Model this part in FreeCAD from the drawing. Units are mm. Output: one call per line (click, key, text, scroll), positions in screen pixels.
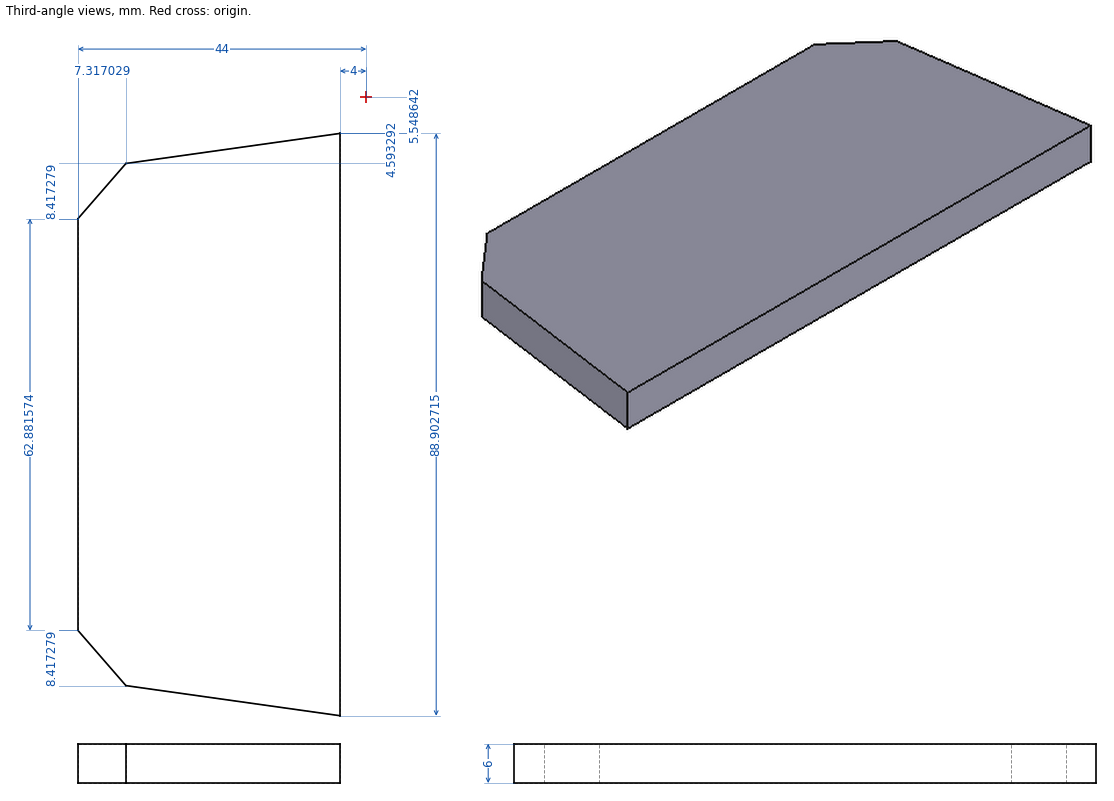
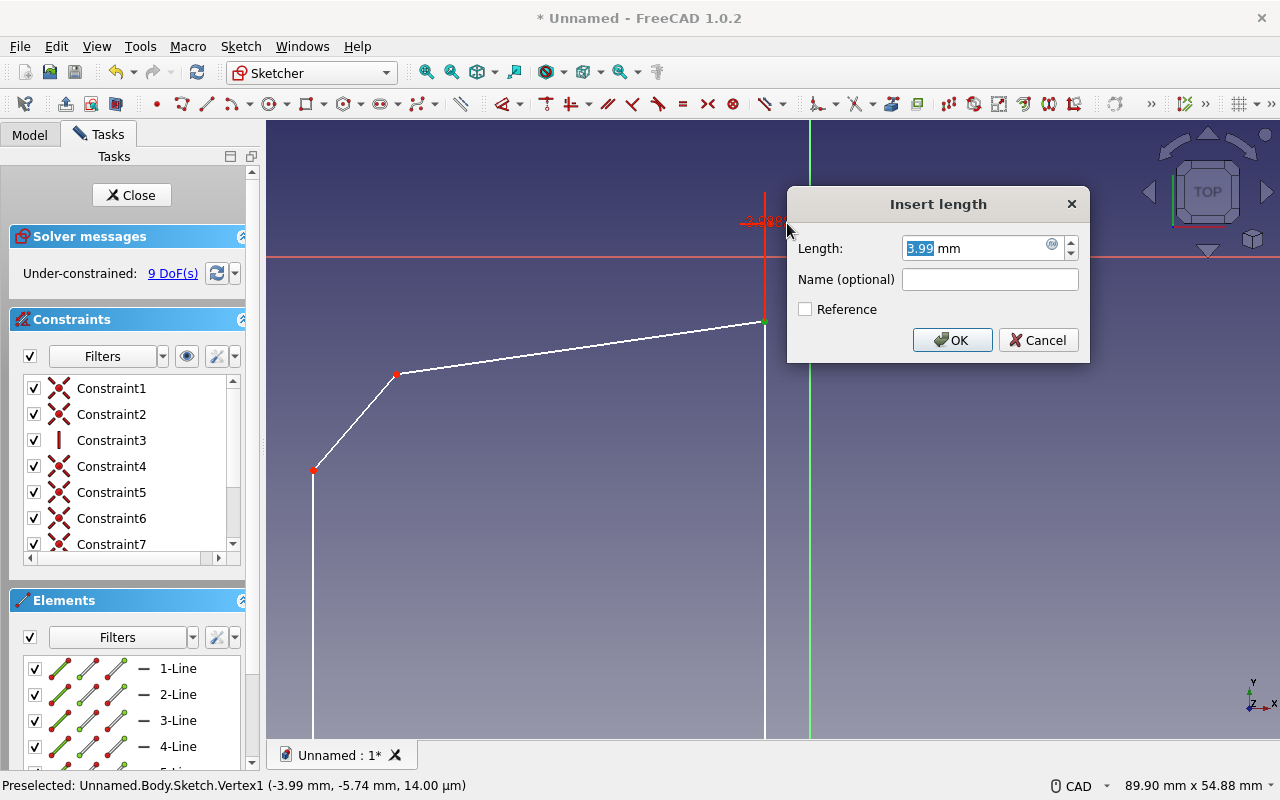
text(4)
key(Return)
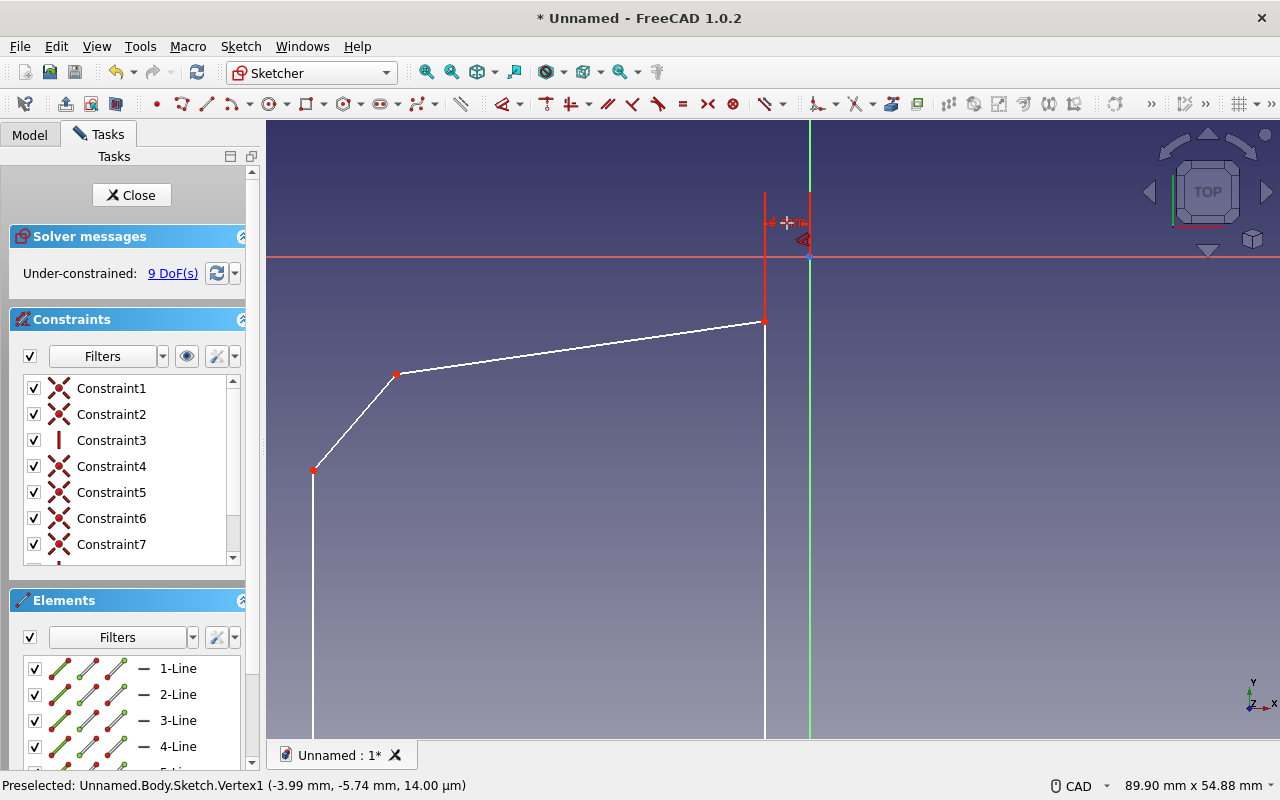
click(313, 471)
click(562, 223)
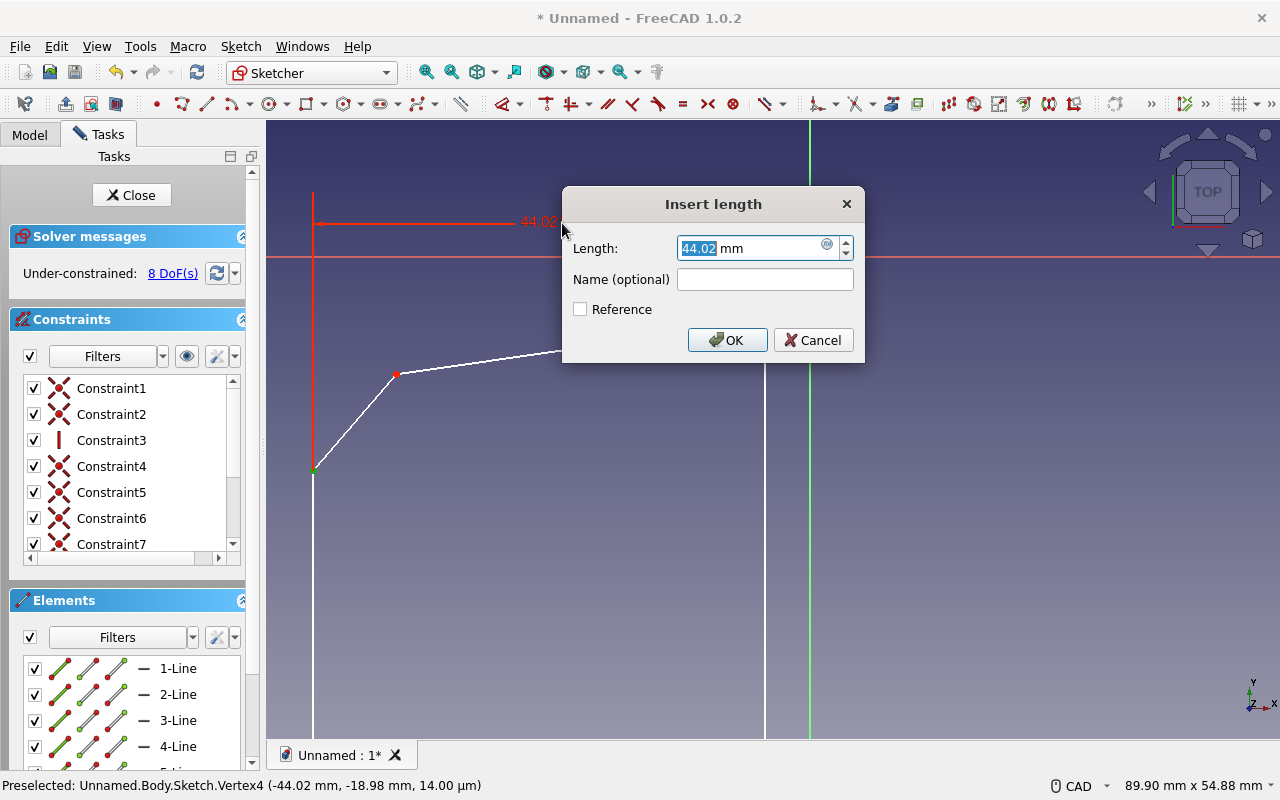
text(44)
key(Return)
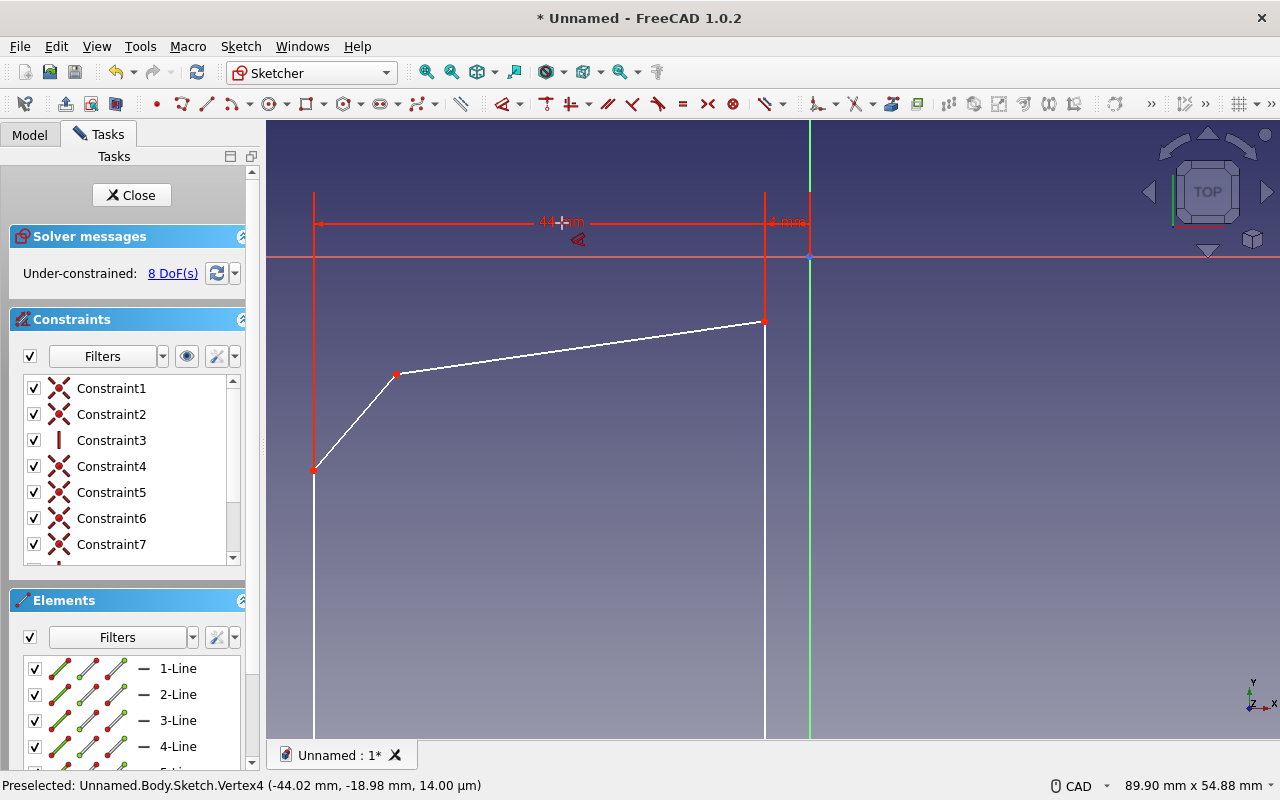
click(314, 683)
click(348, 591)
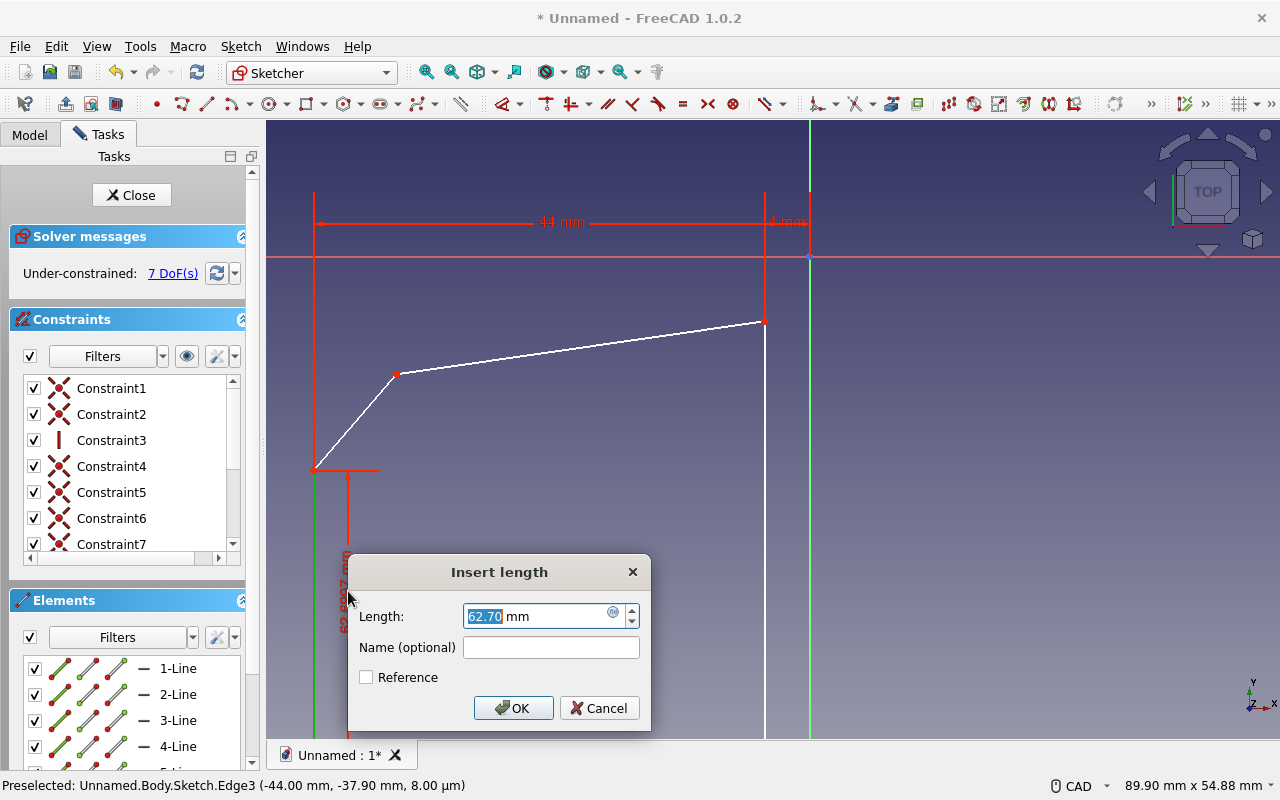
text(62.881574)
key(Return)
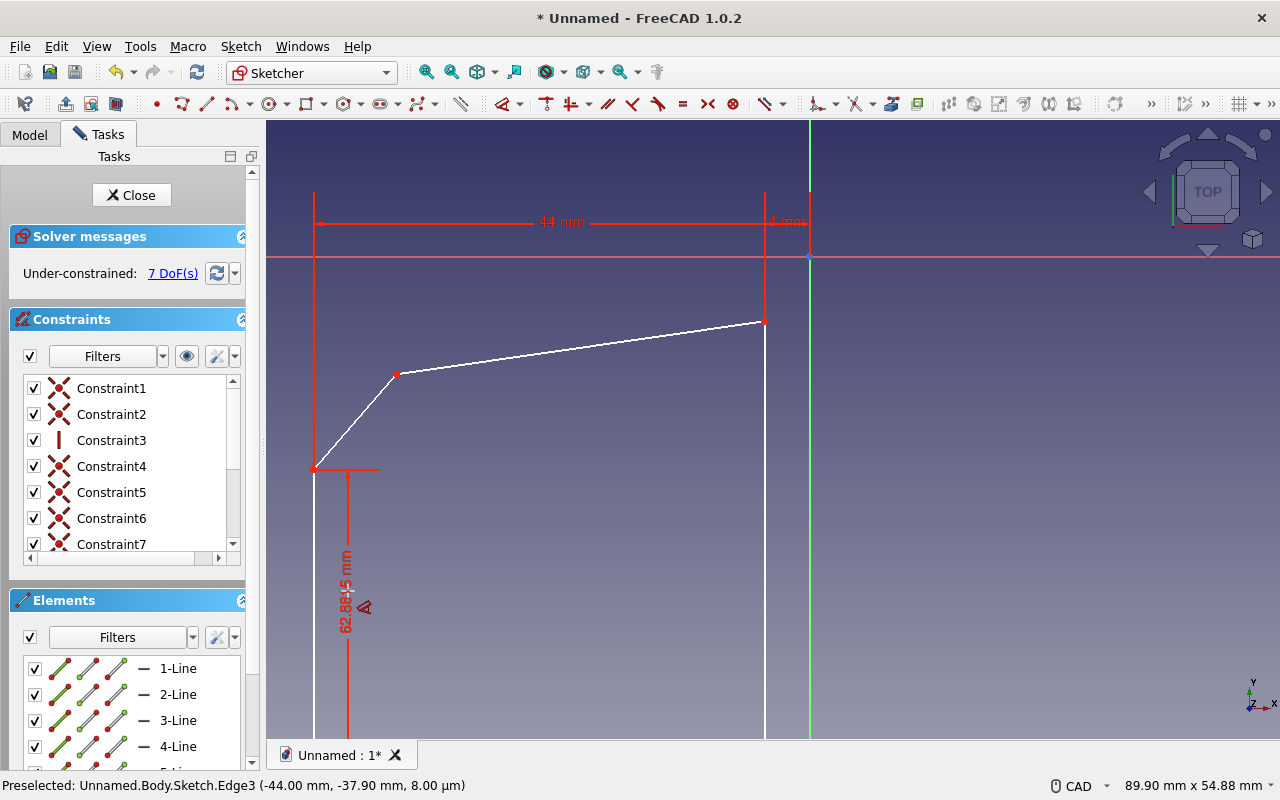
click(765, 622)
click(731, 516)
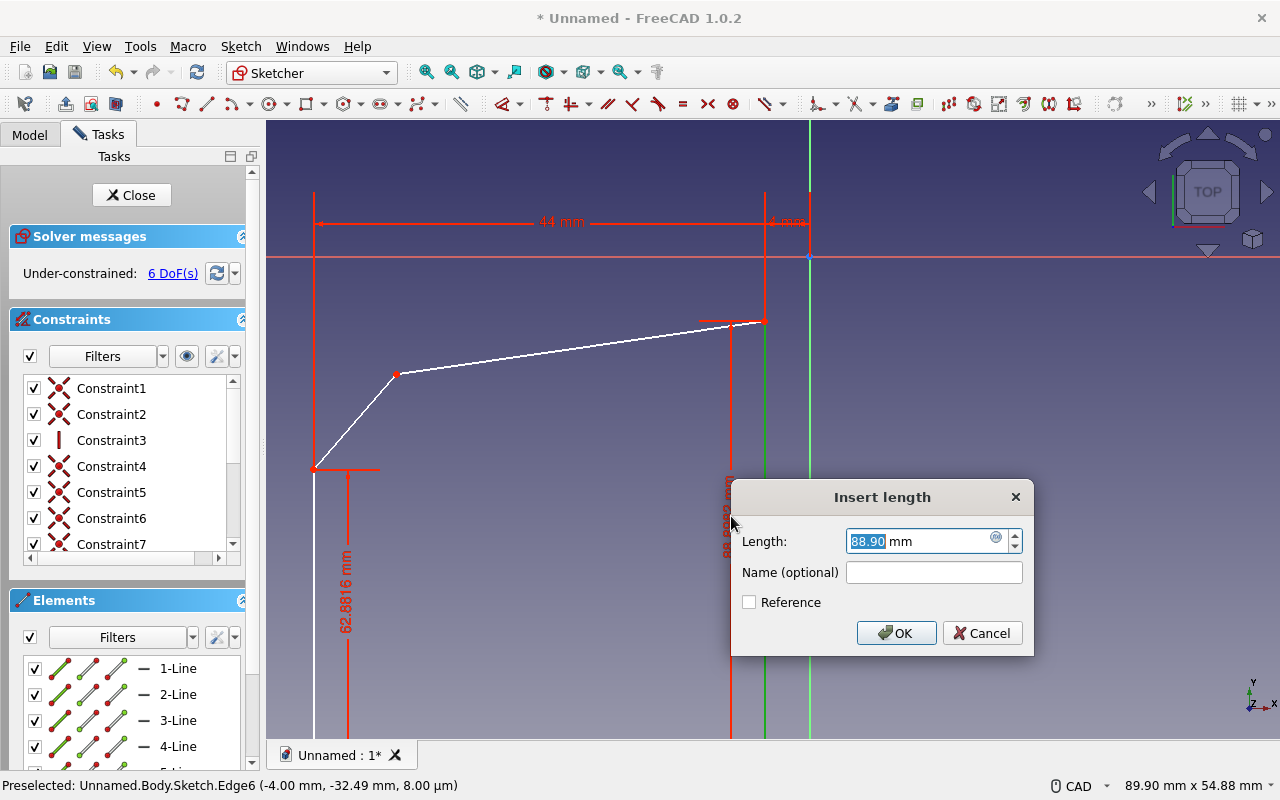
text(88.902715)
key(Return)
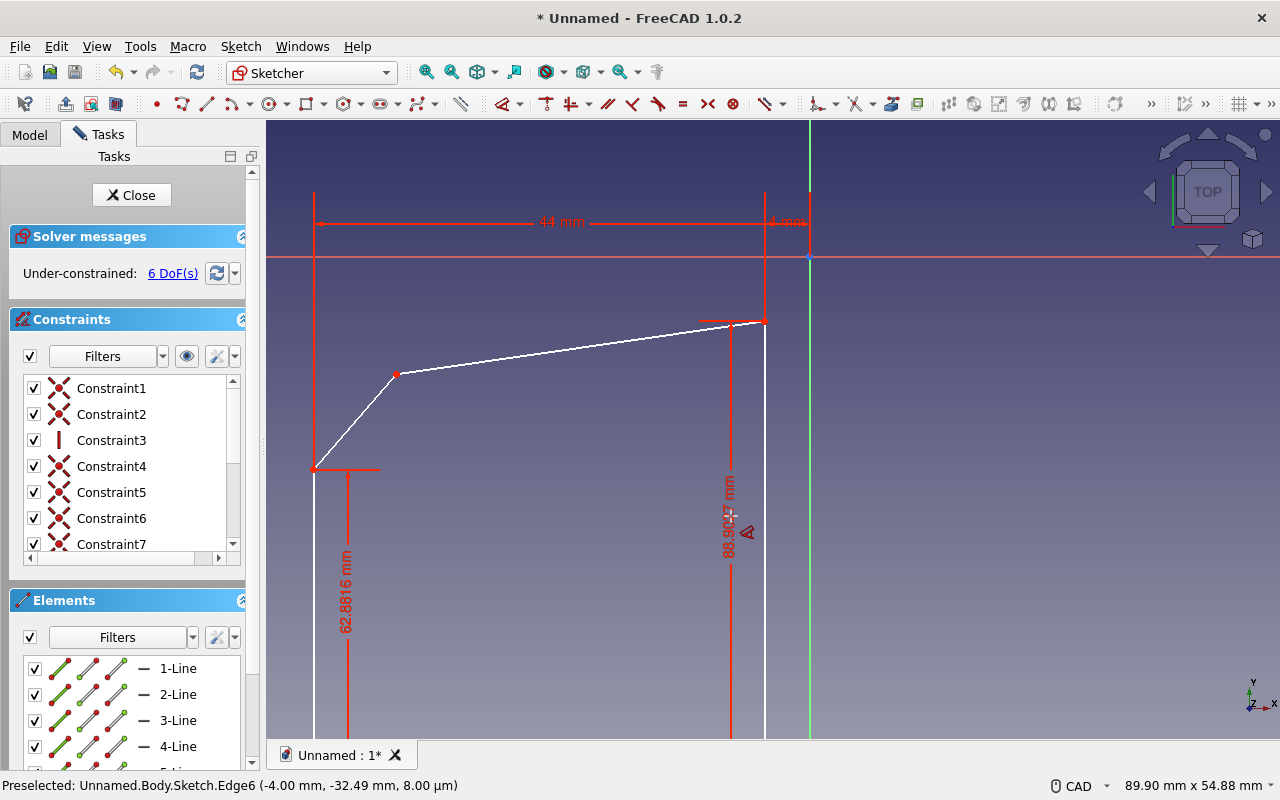
click(765, 321)
click(844, 289)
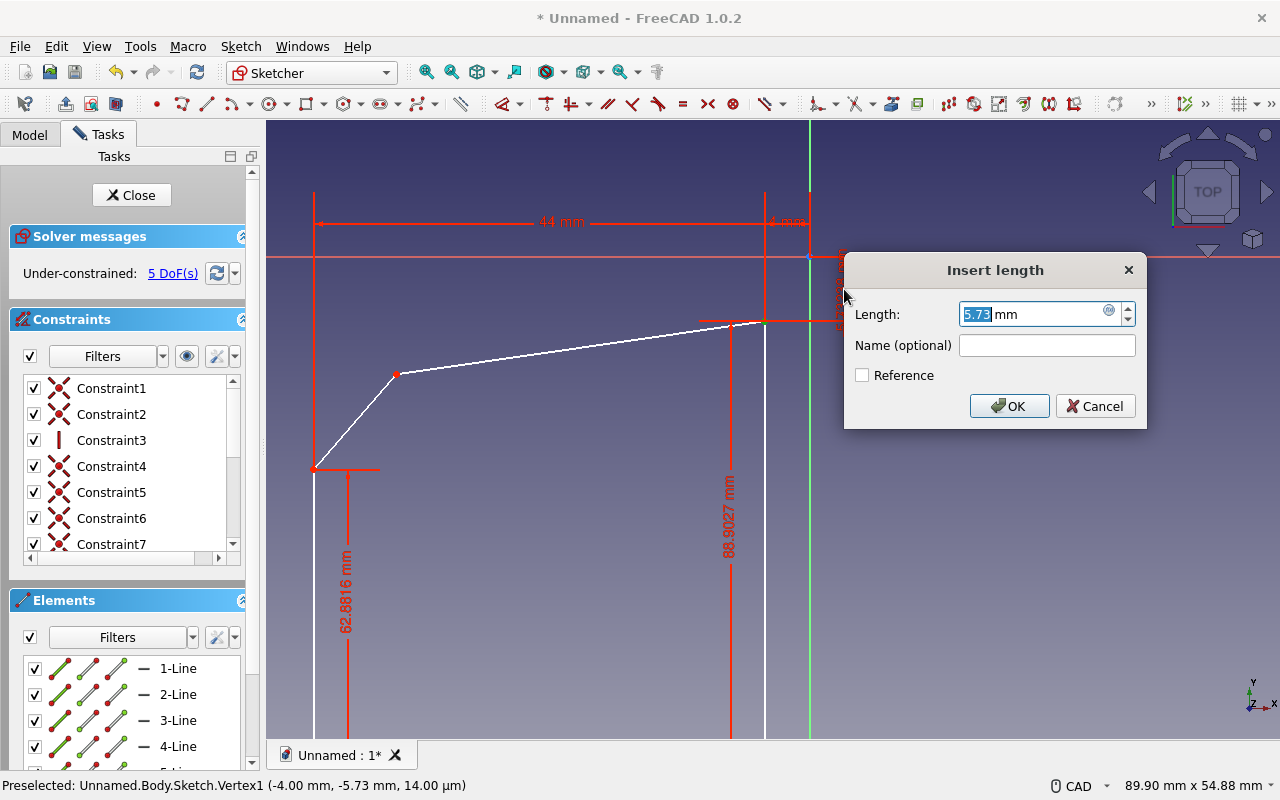
text(5.548642)
key(Return)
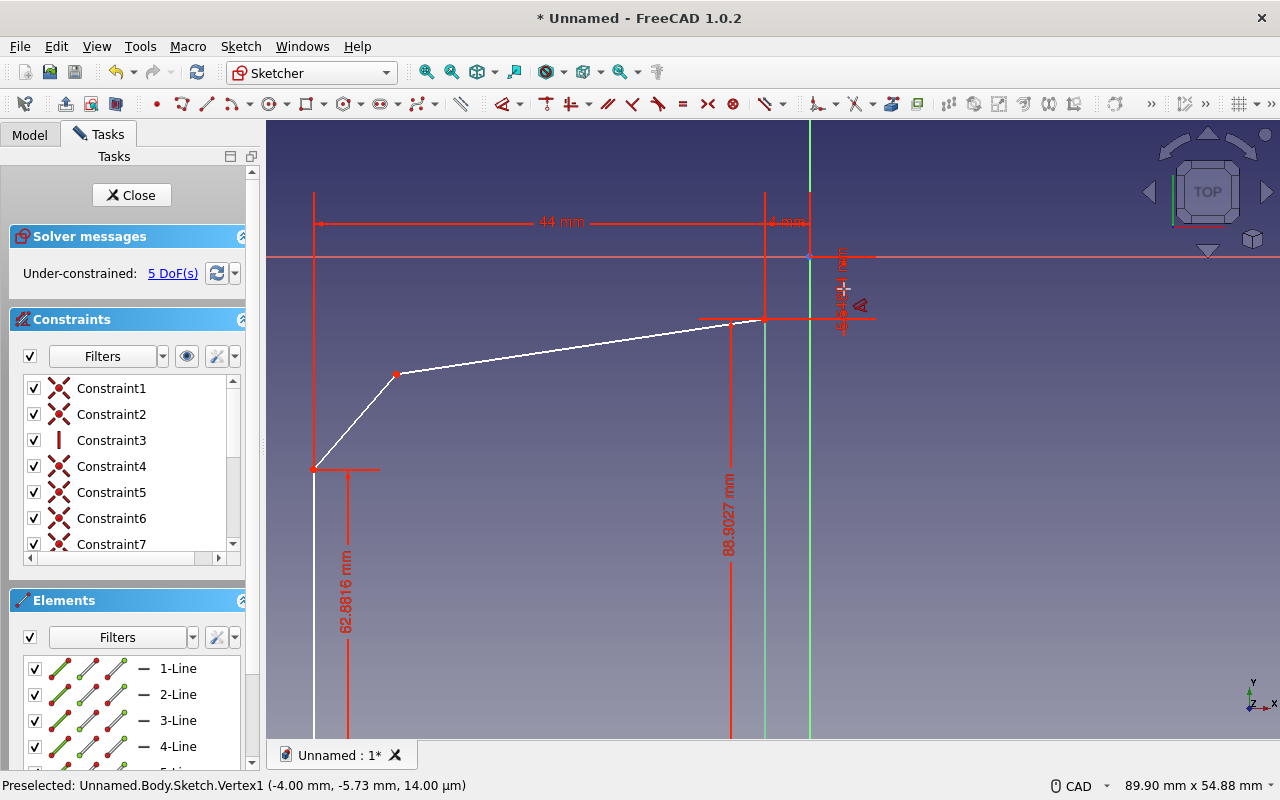
click(654, 336)
click(362, 347)